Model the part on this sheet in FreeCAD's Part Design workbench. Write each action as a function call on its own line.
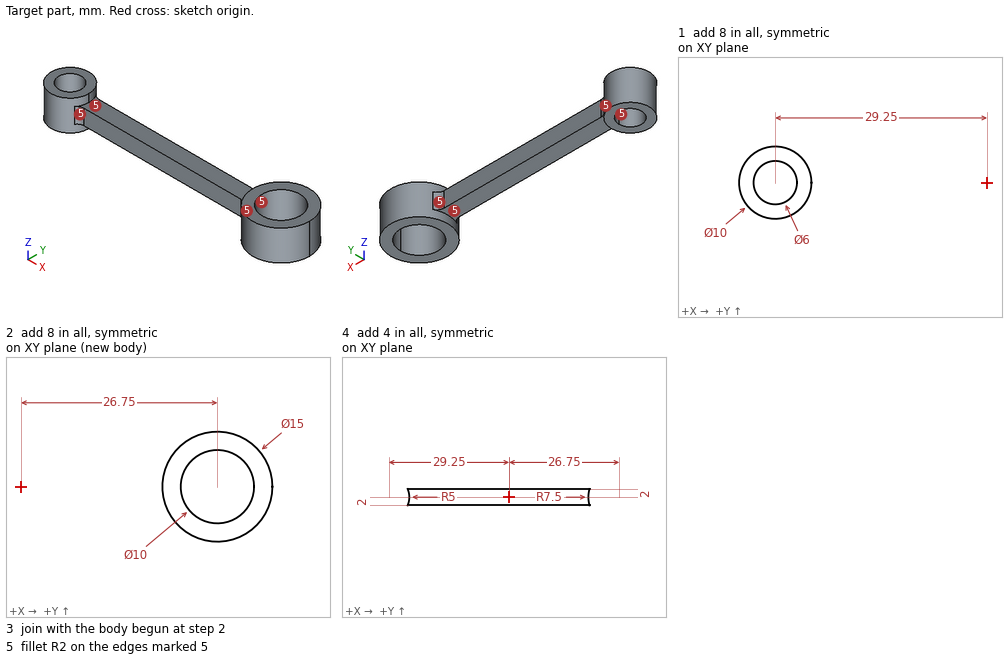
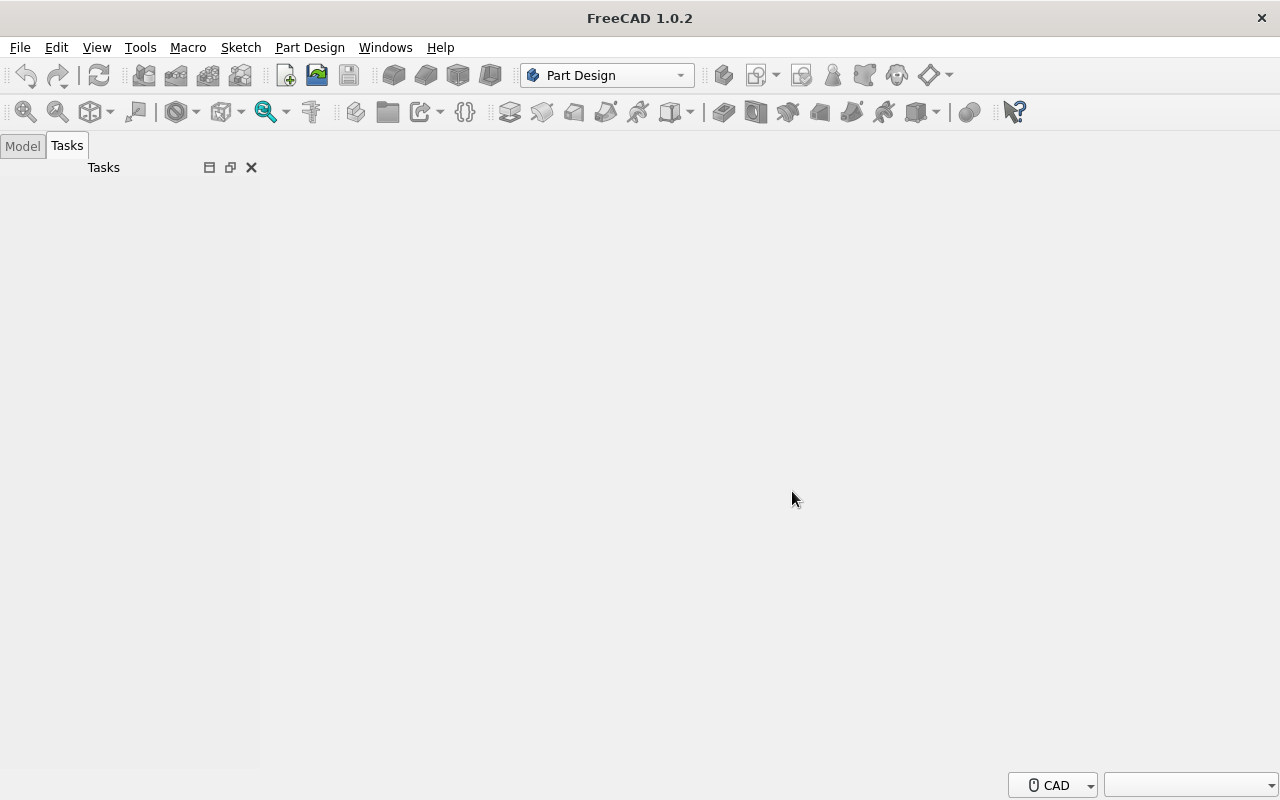
click(286, 76)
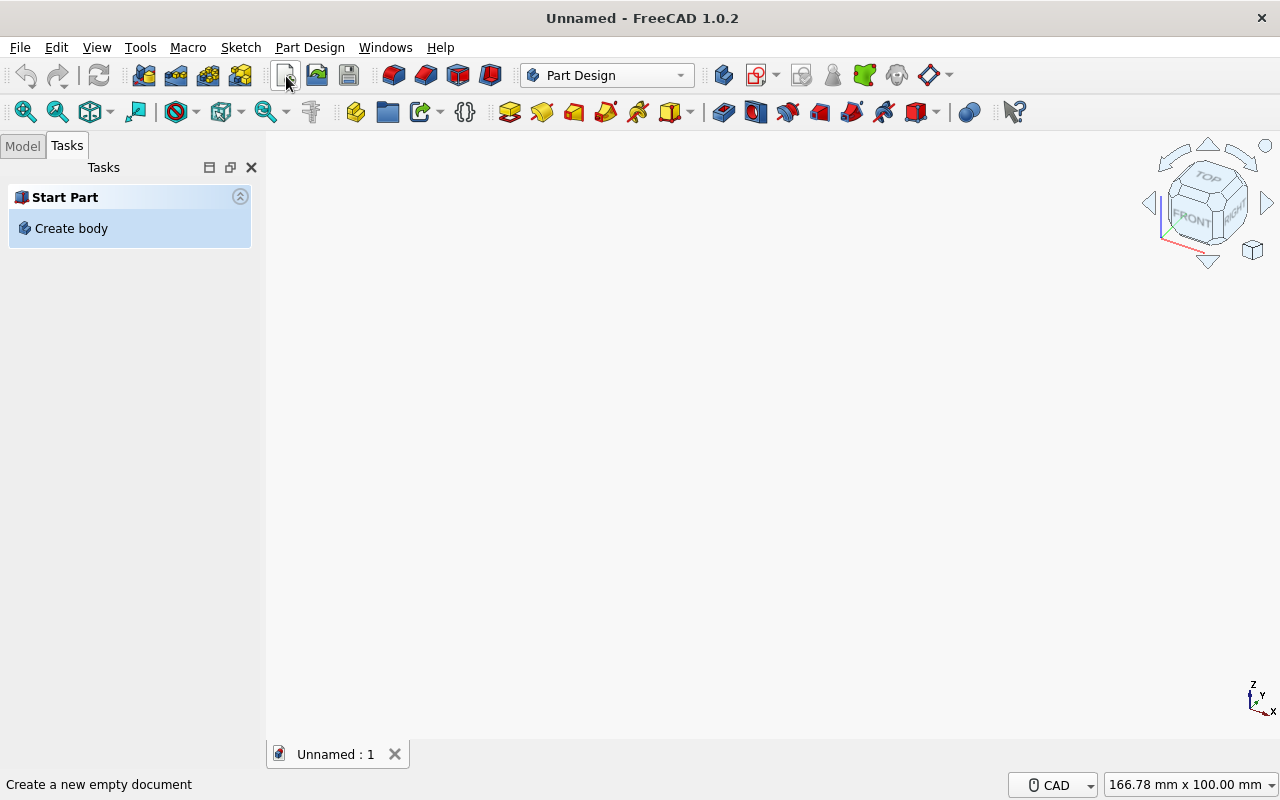
click(756, 76)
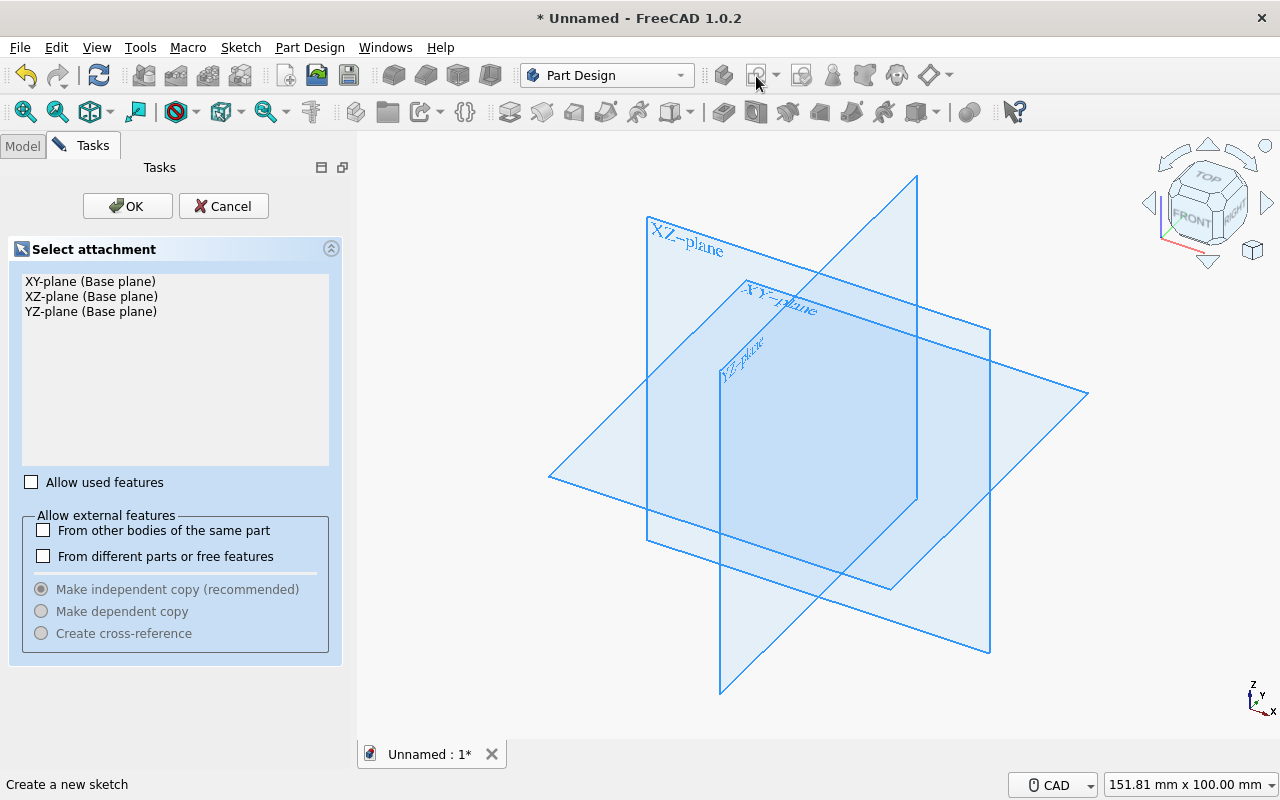
click(82, 282)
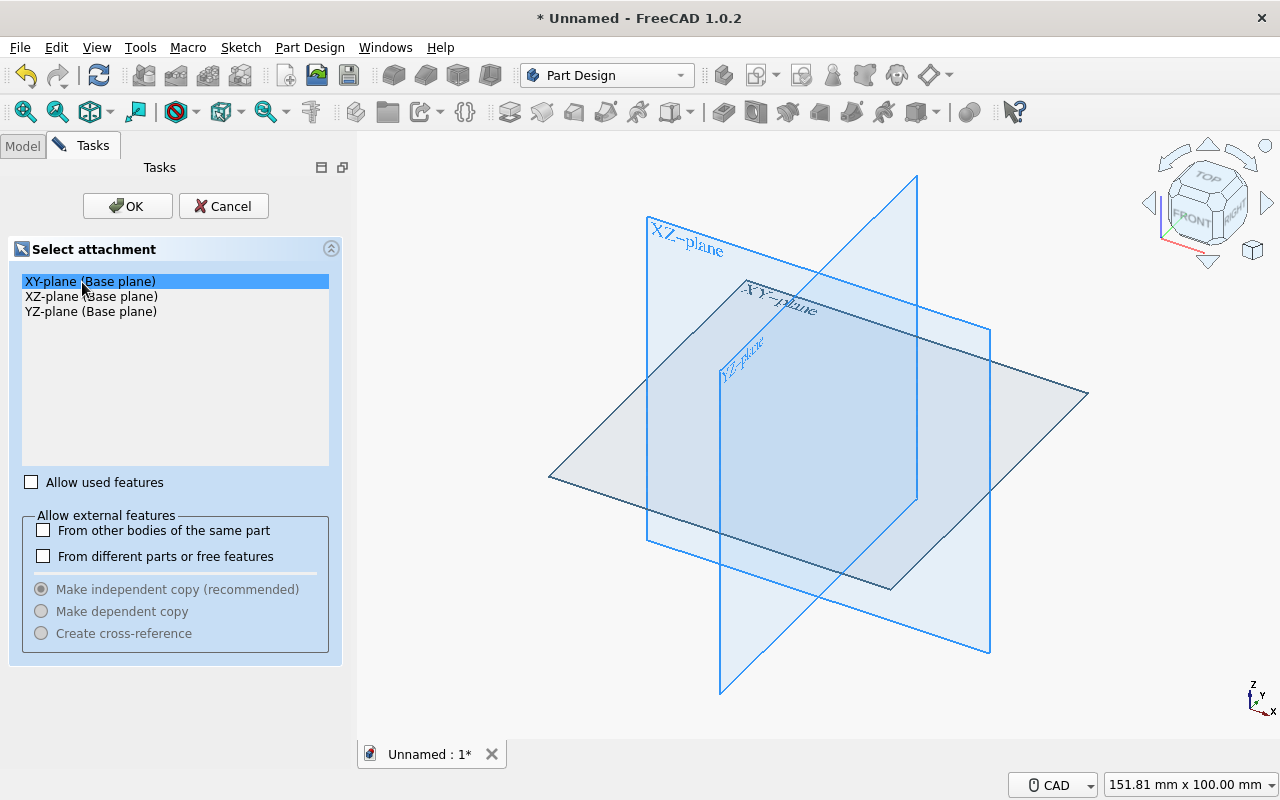
click(128, 206)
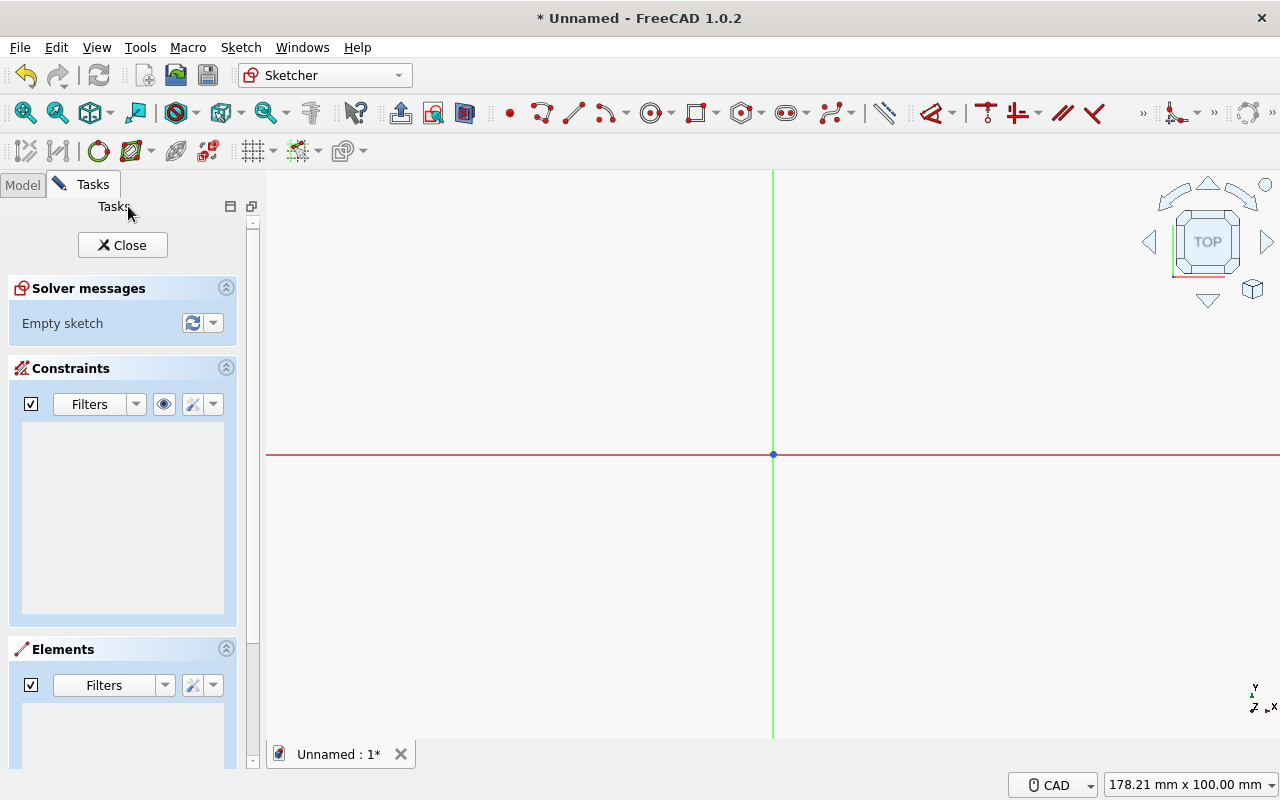
scroll(587, 455, up, 9)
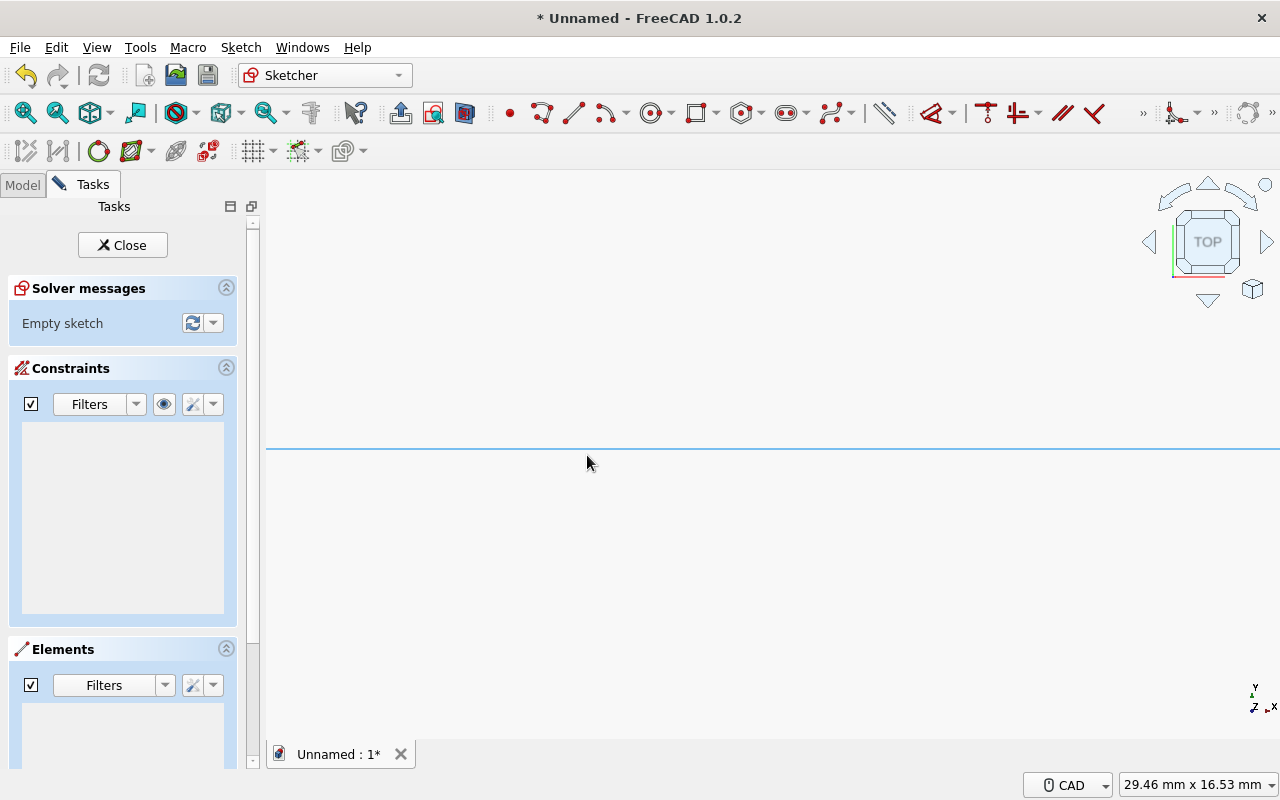
key(g)
key(c)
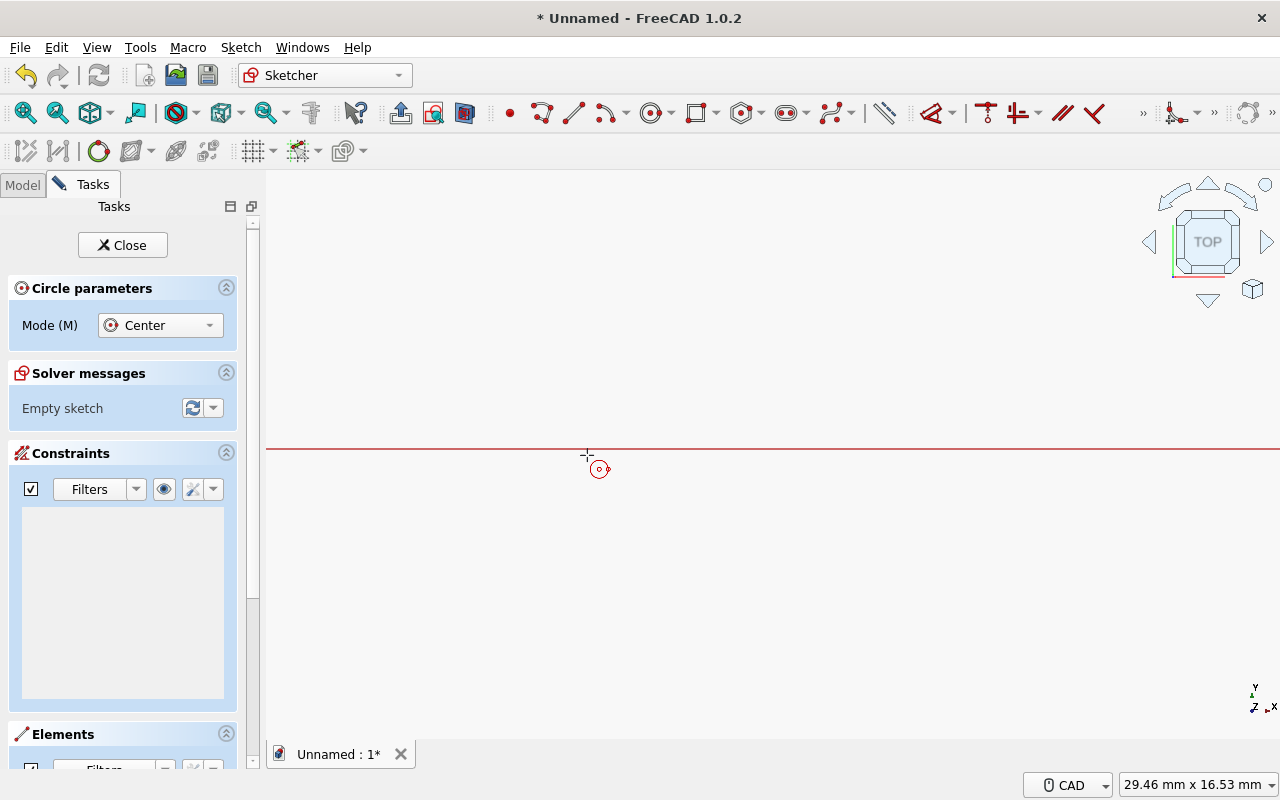
click(704, 449)
click(825, 328)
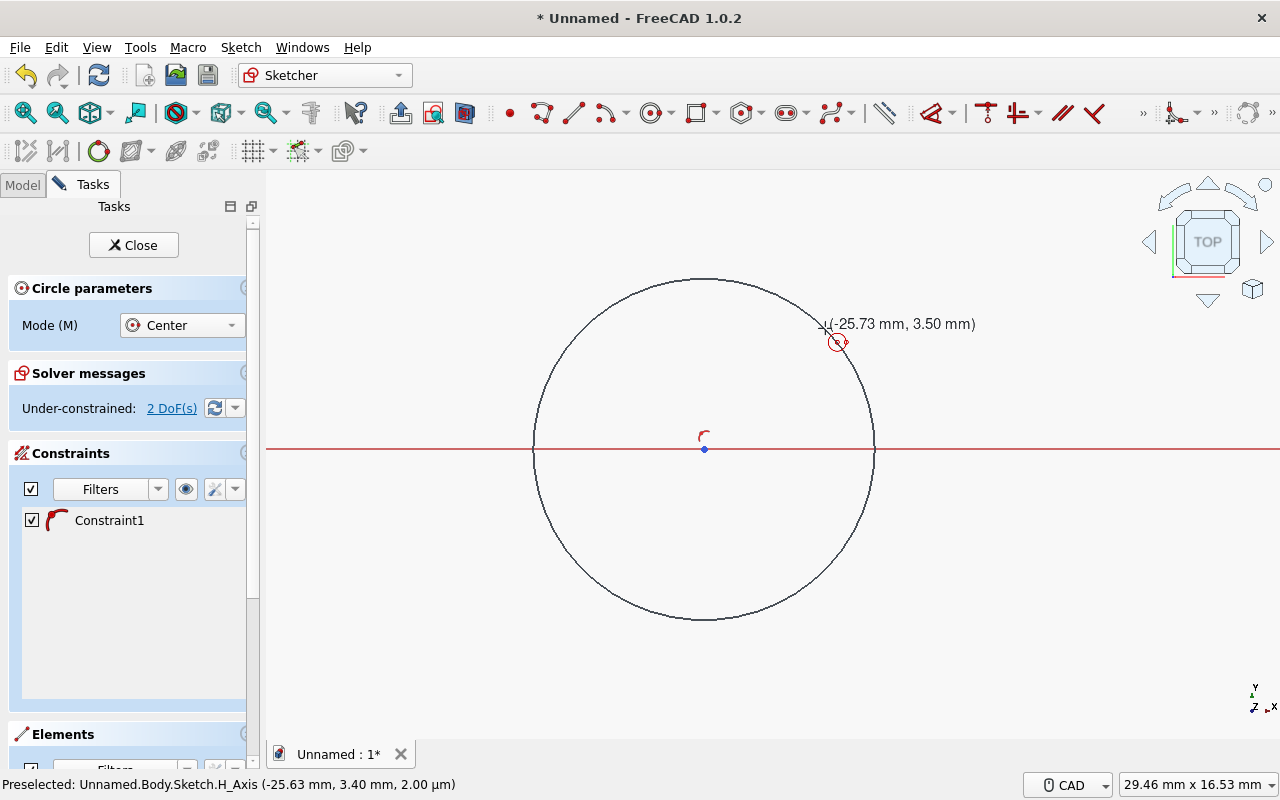
click(704, 449)
click(777, 376)
key(Escape)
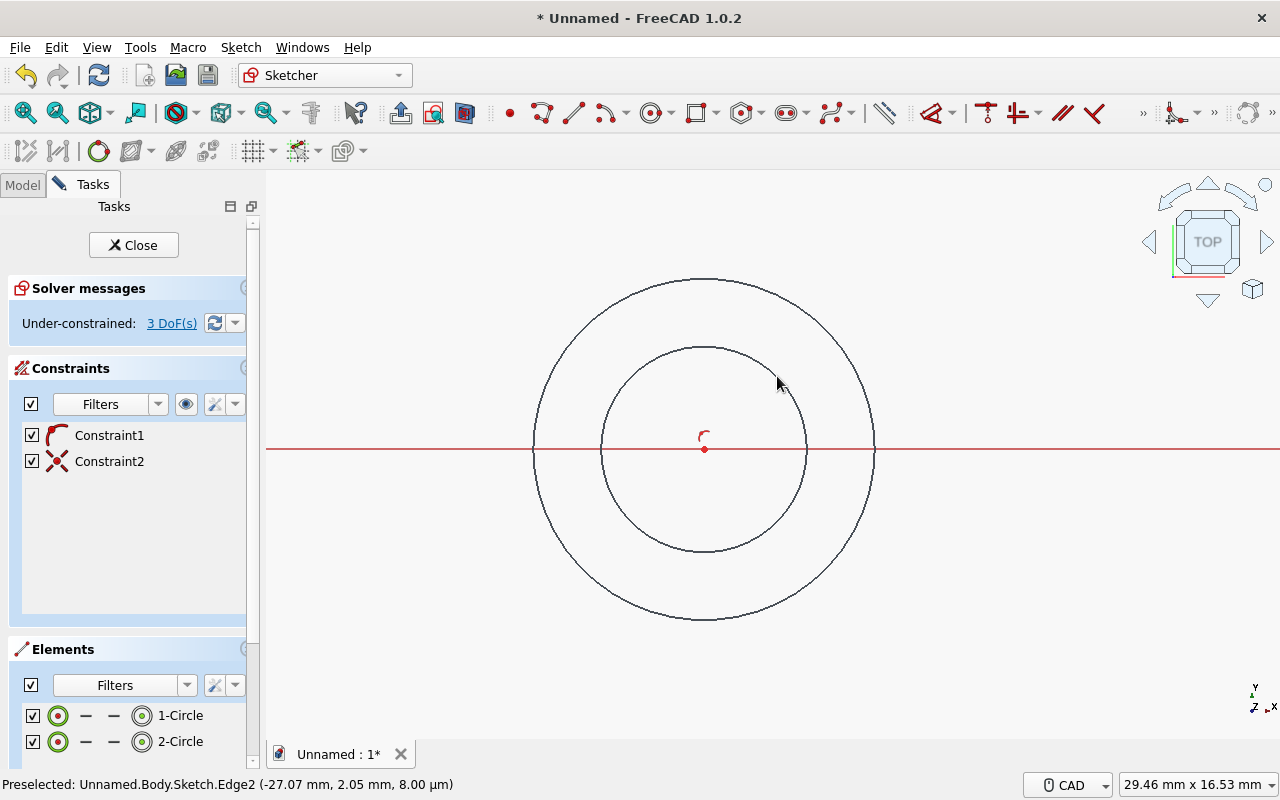
key(d)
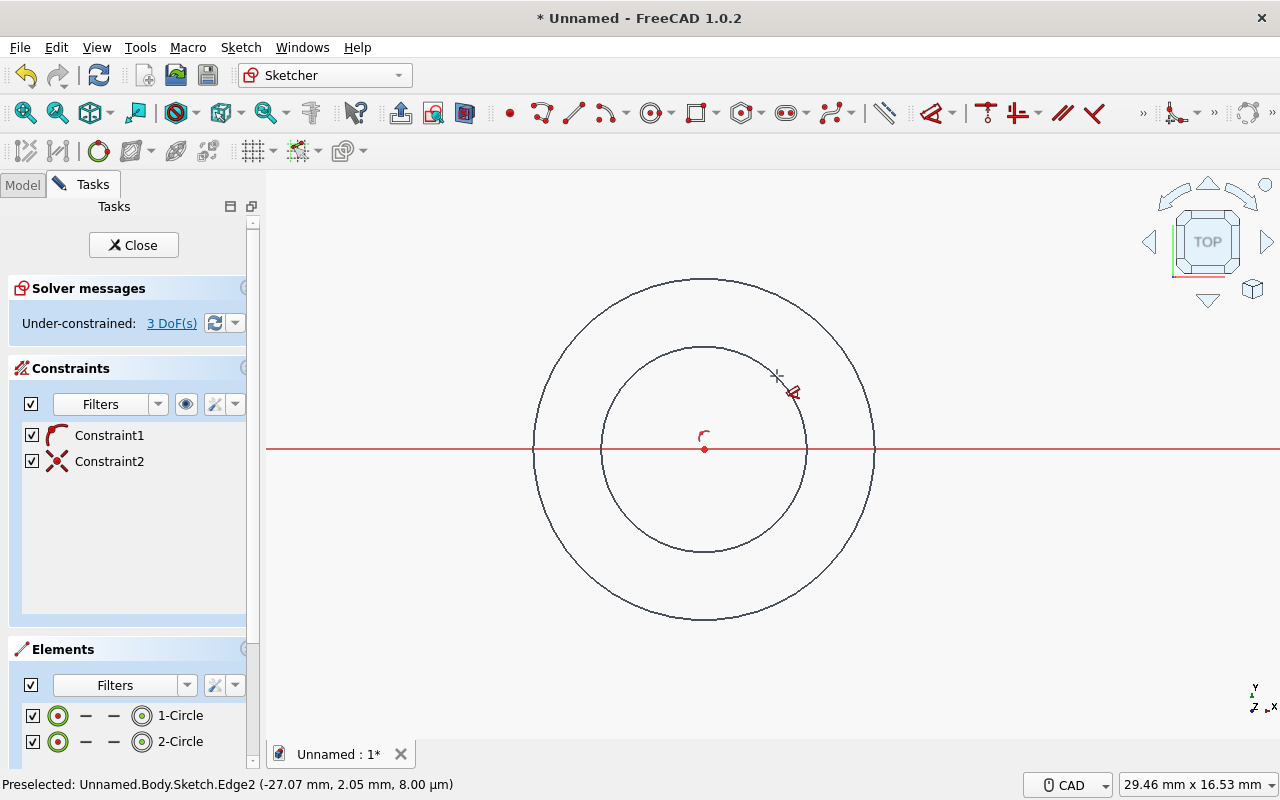
click(824, 328)
click(846, 305)